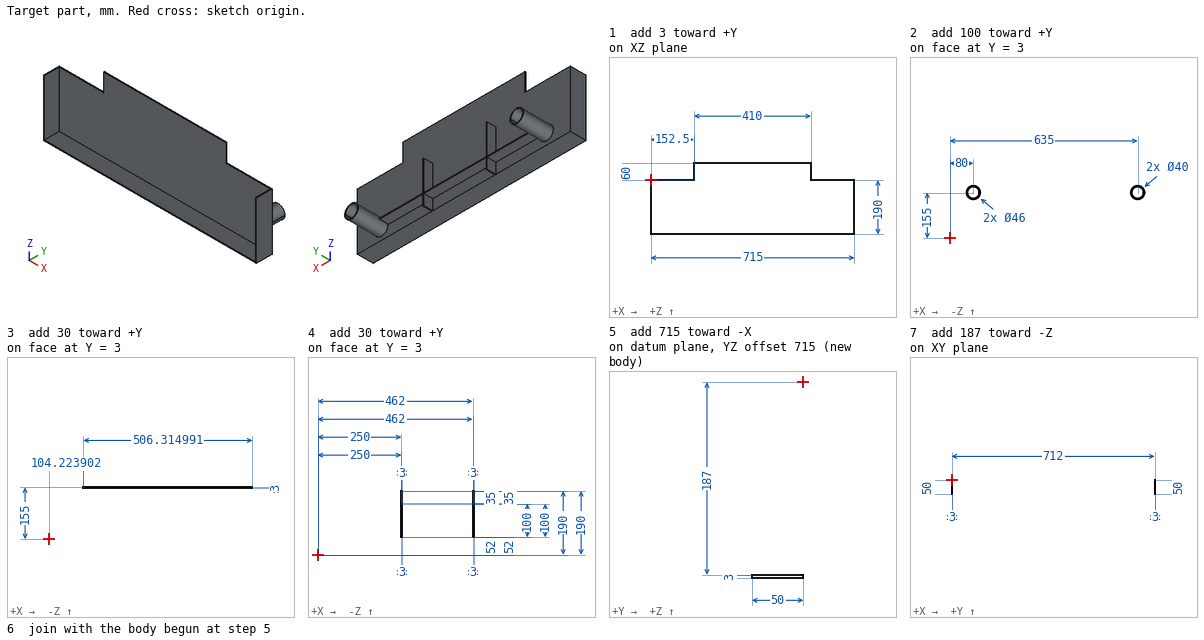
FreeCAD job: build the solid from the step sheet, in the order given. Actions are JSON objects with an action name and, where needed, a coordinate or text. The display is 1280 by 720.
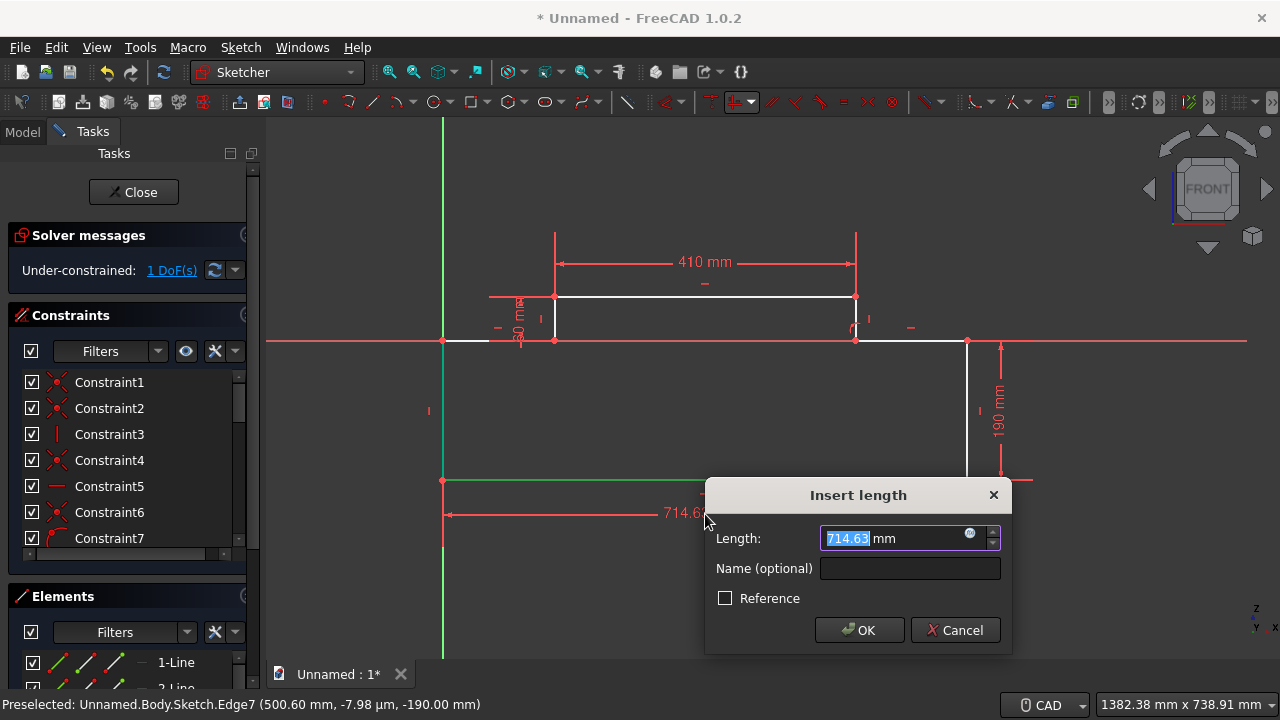
{"action": "type", "text": "715"}
{"action": "key", "text": "Return"}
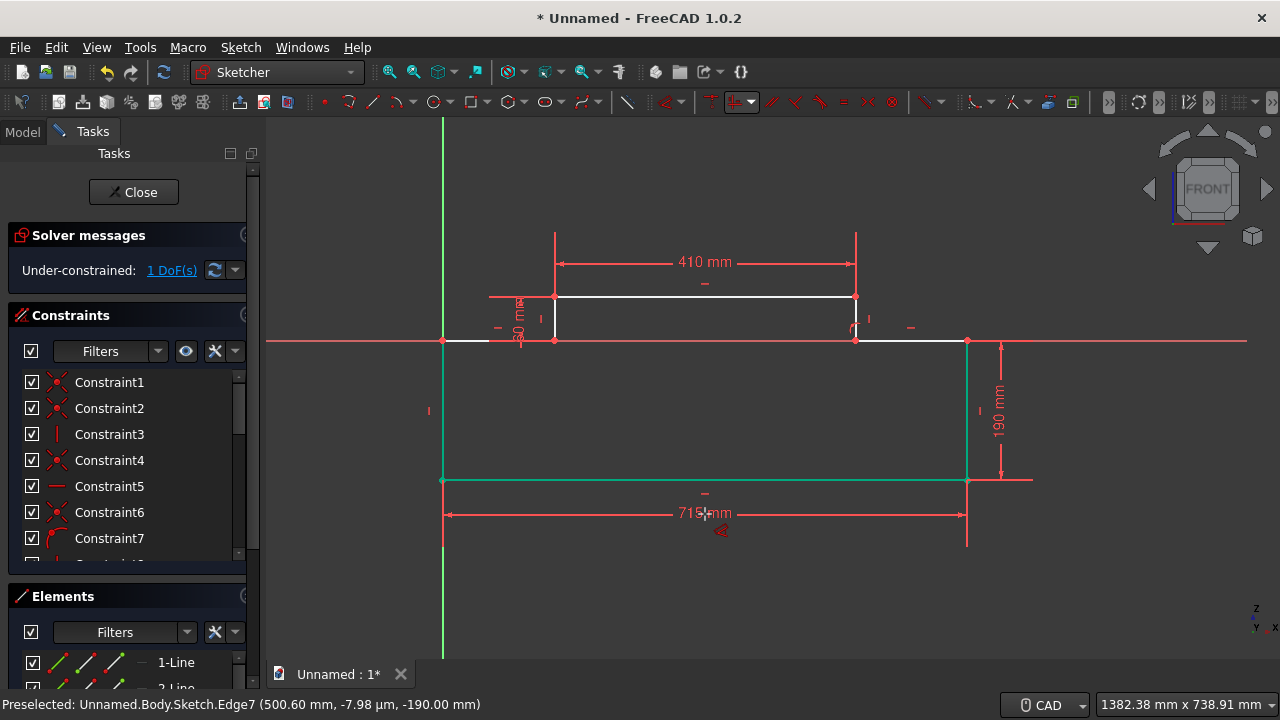
{"action": "left_click", "coordinate": [476, 341]}
{"action": "left_click", "coordinate": [499, 375]}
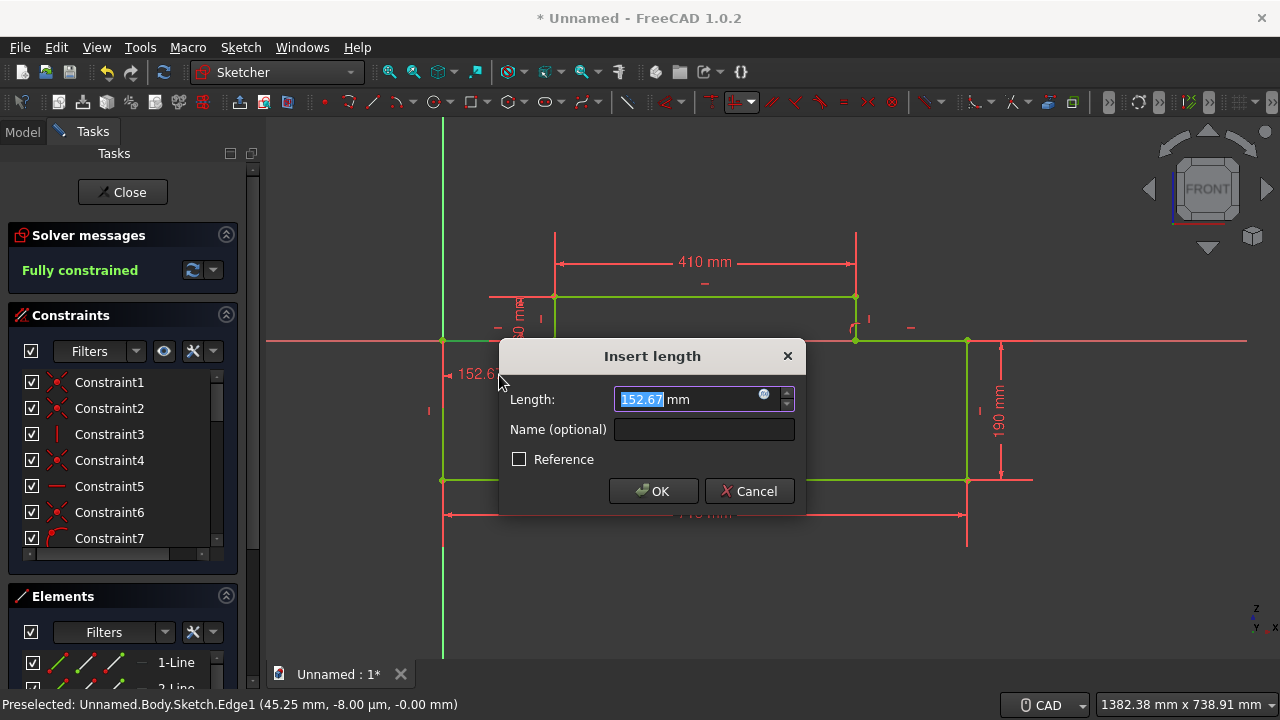
{"action": "type", "text": "152.5"}
{"action": "key", "text": "Return"}
{"action": "key", "text": "Escape"}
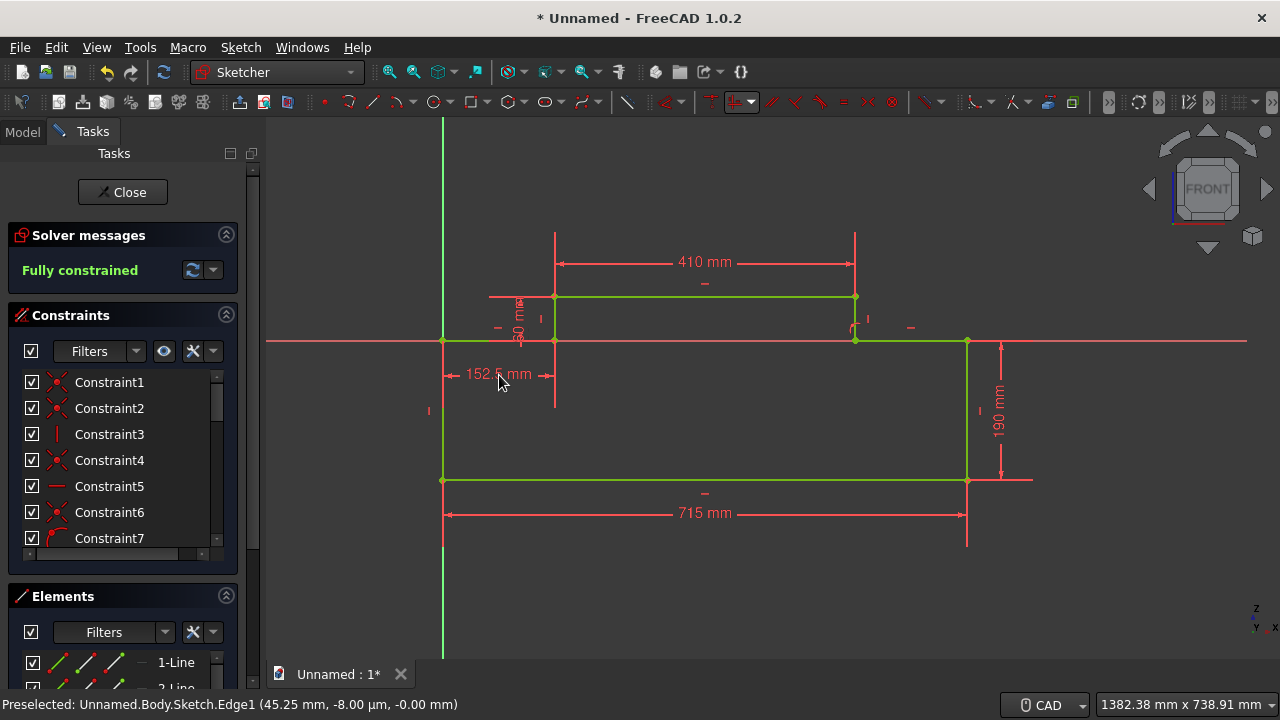
{"action": "left_click", "coordinate": [123, 192]}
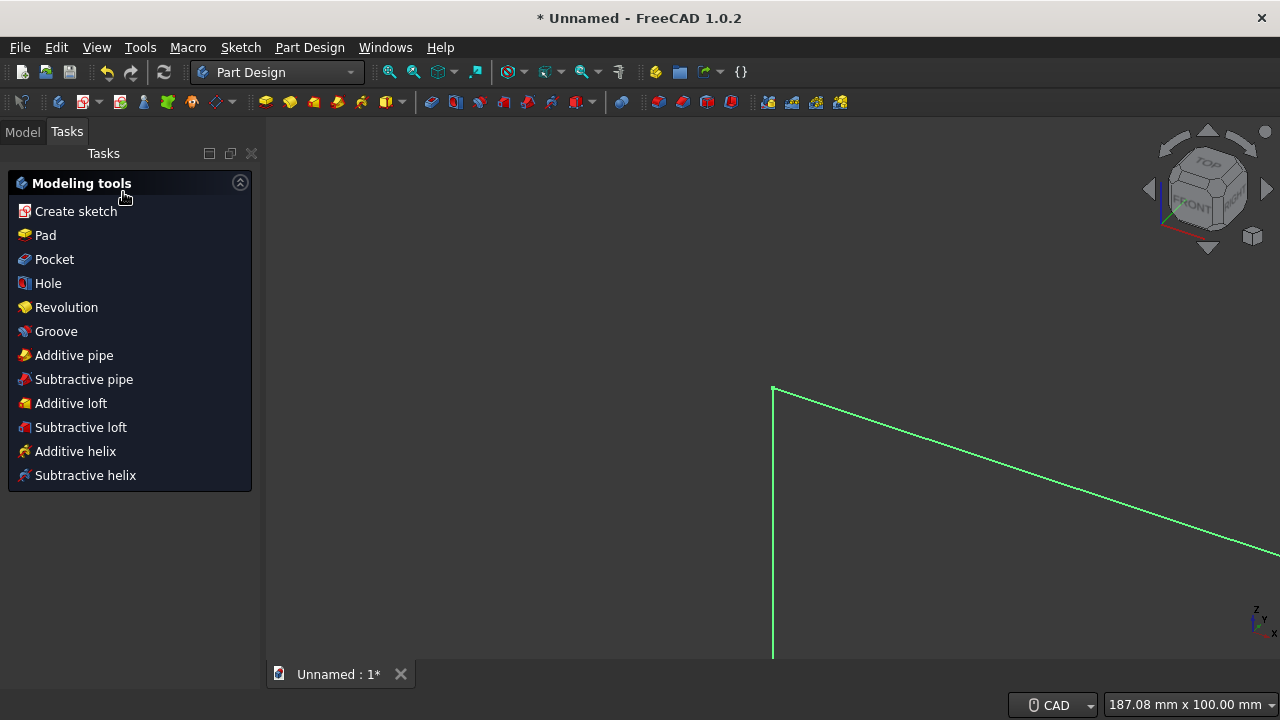
{"action": "left_click", "coordinate": [266, 102]}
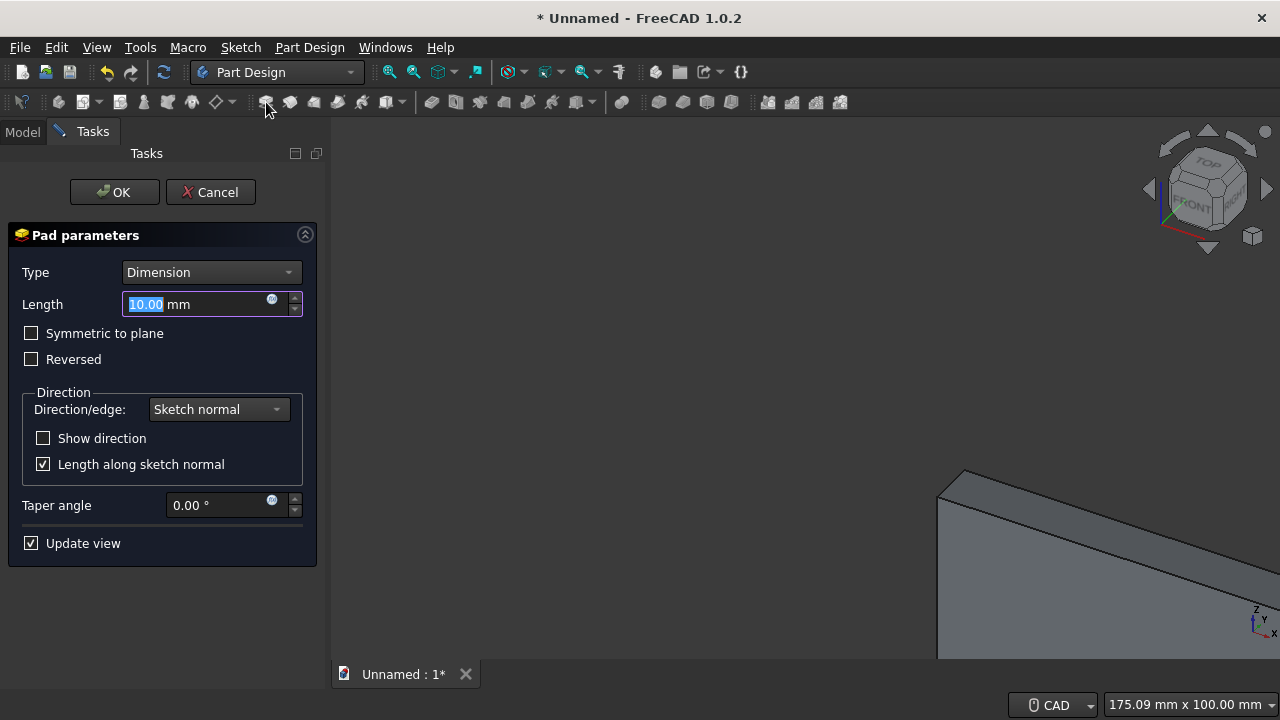
{"action": "type", "text": "3"}
{"action": "key", "text": "Tab"}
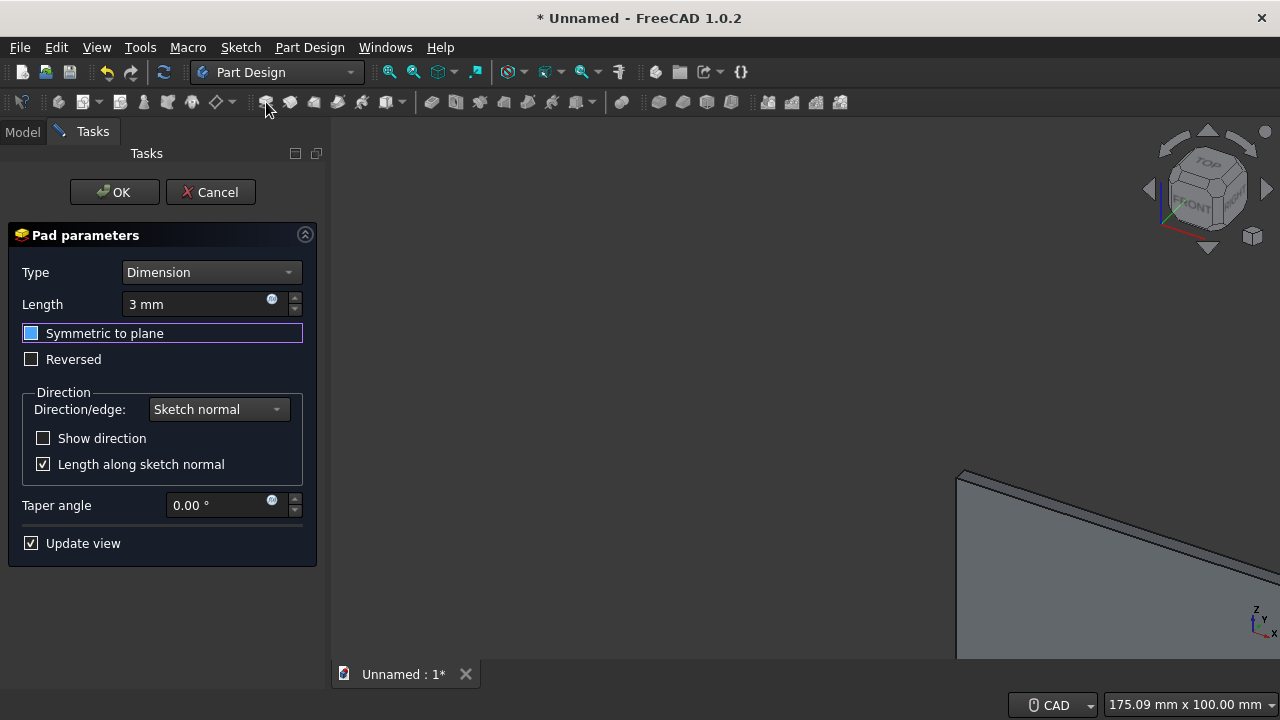
{"action": "left_click", "coordinate": [30, 359]}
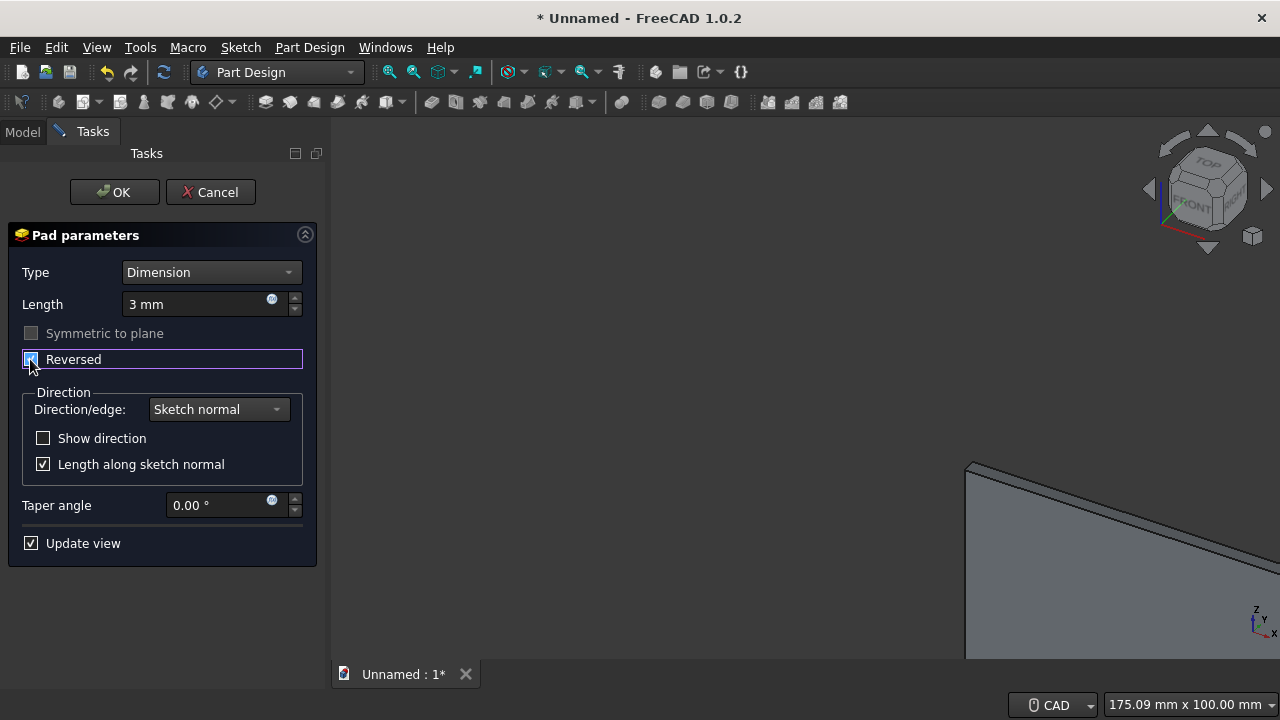
{"action": "left_click", "coordinate": [115, 192]}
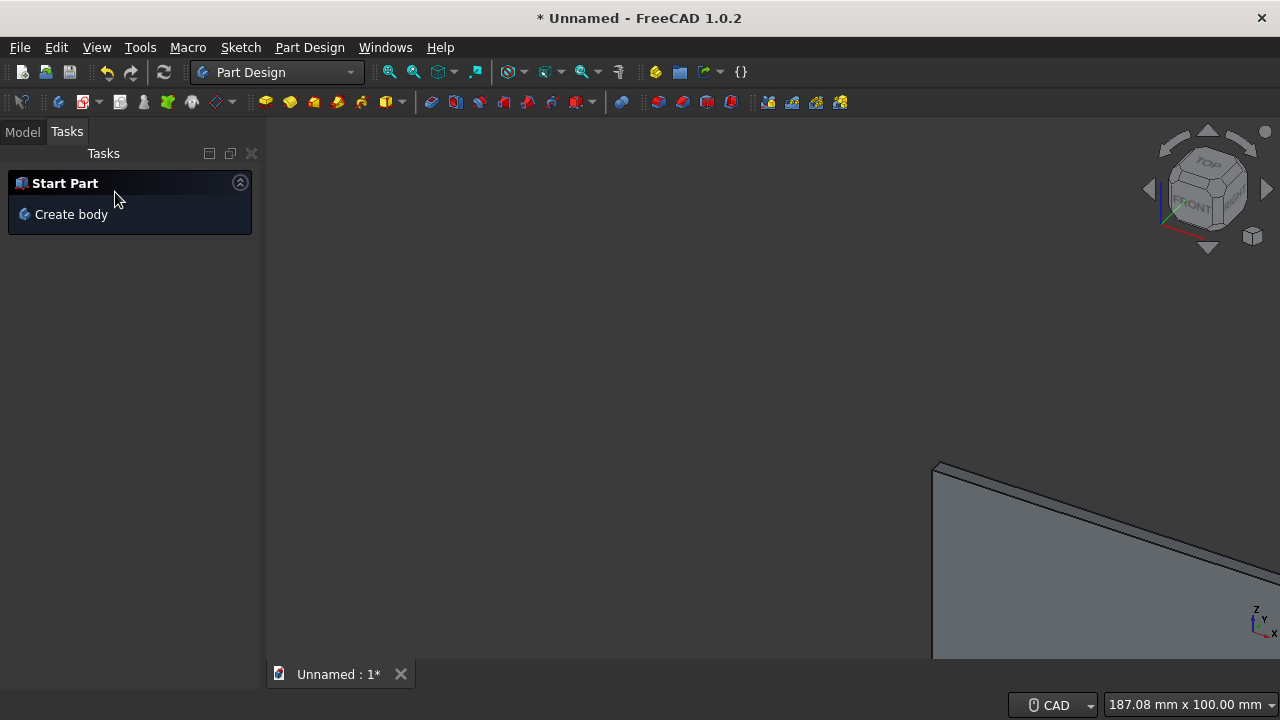
{"action": "left_click", "coordinate": [390, 72]}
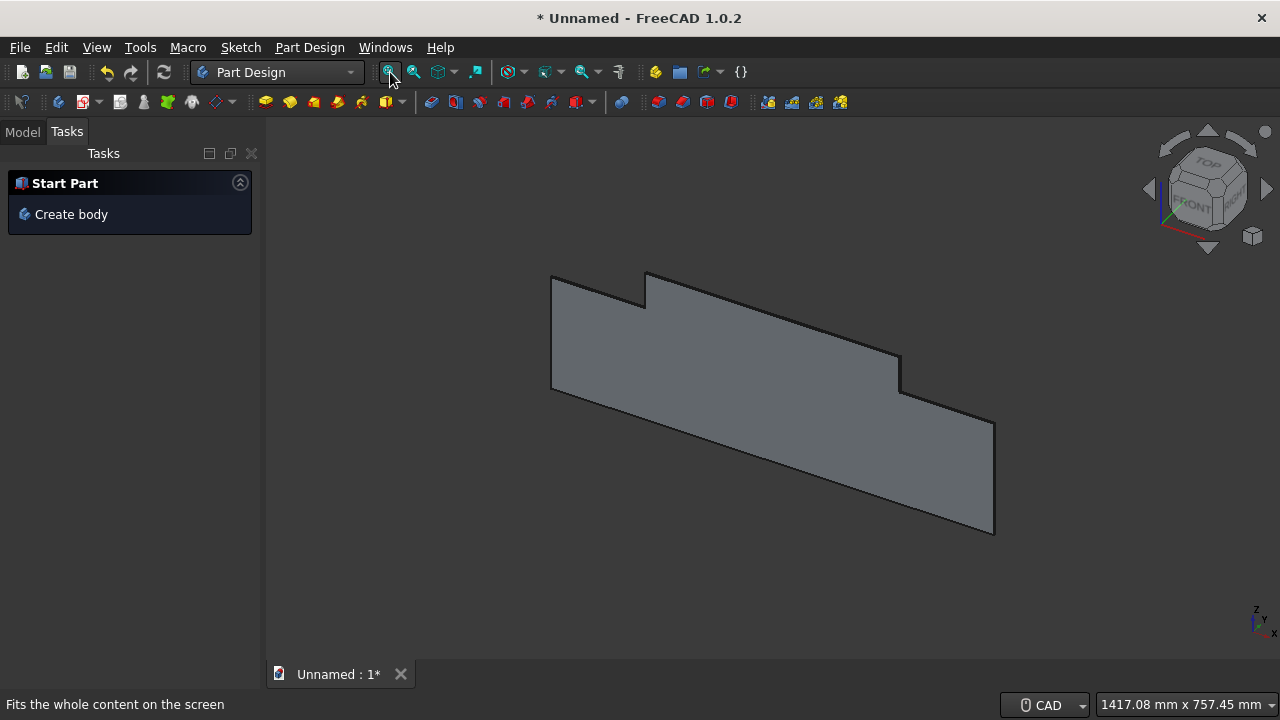
{"action": "key", "text": "4"}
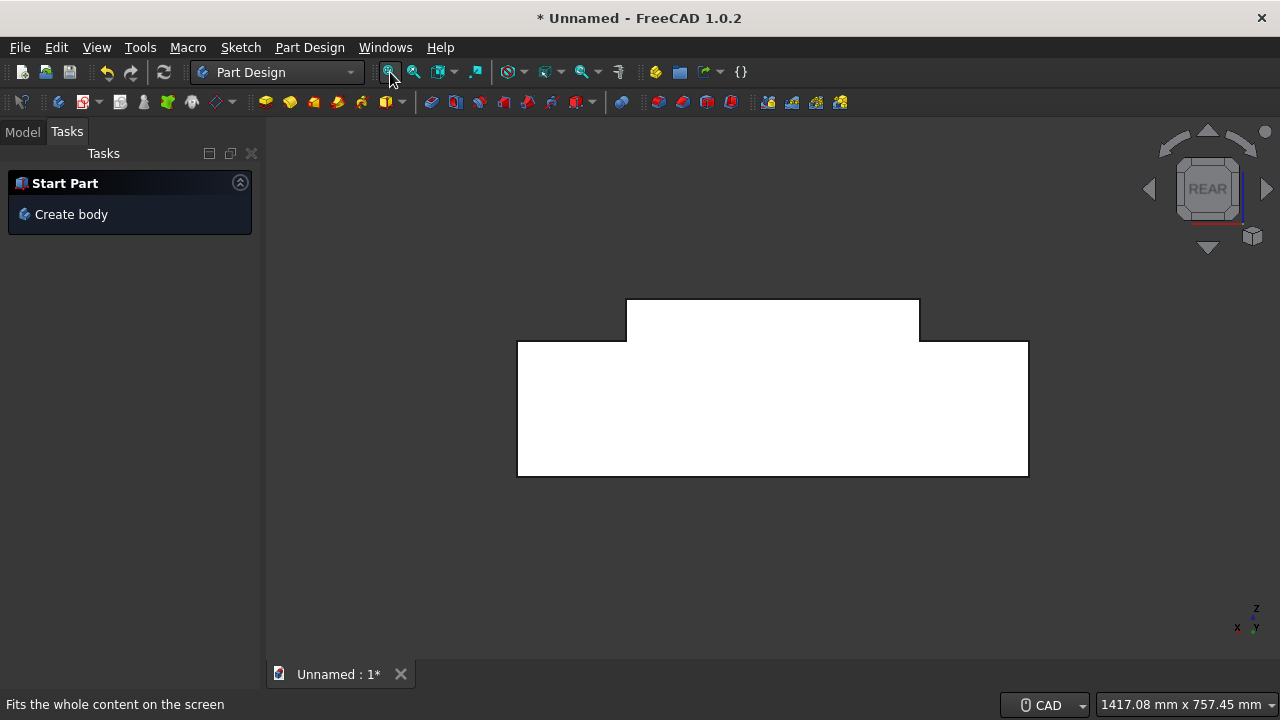
{"action": "left_click", "coordinate": [773, 387]}